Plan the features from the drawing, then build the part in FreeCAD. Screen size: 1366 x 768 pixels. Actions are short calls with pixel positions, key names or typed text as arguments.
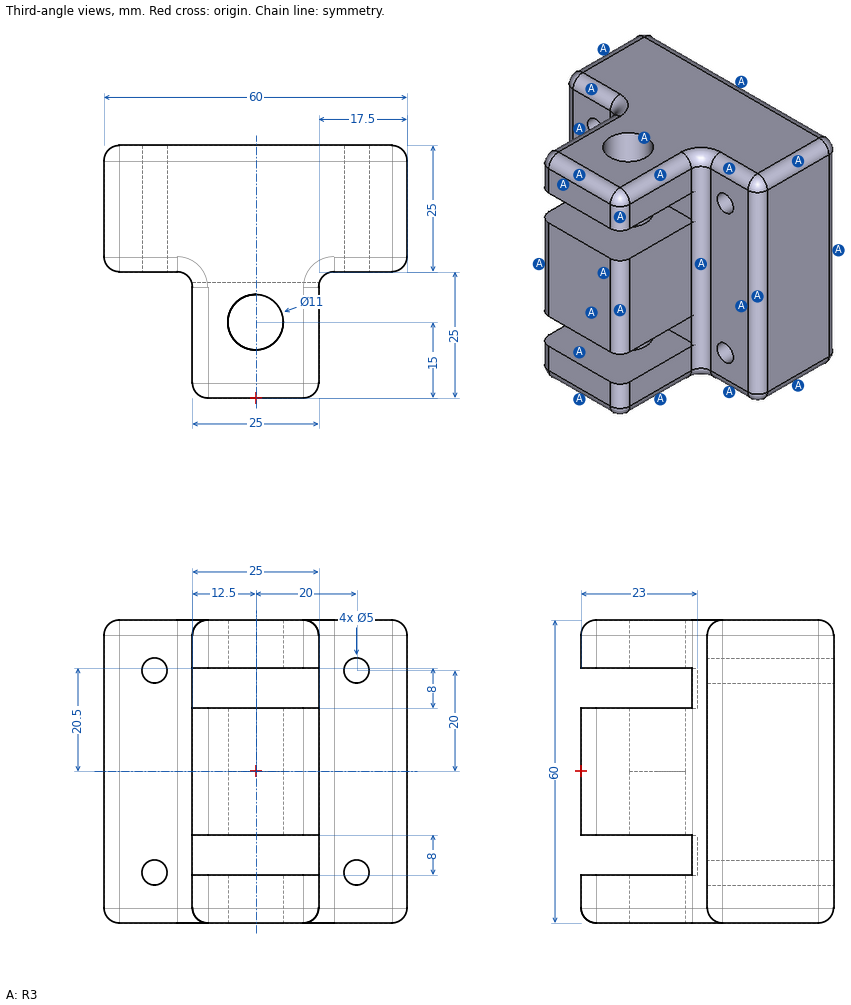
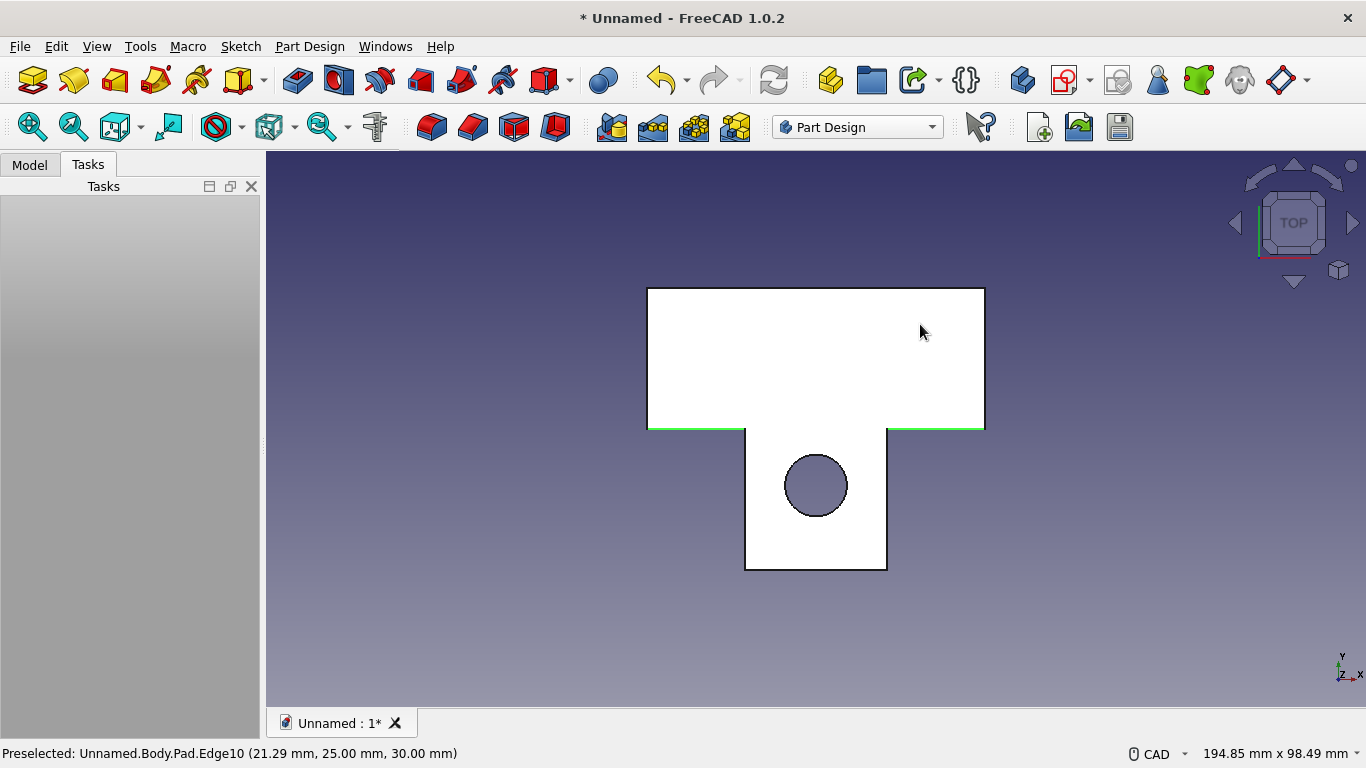
key(1)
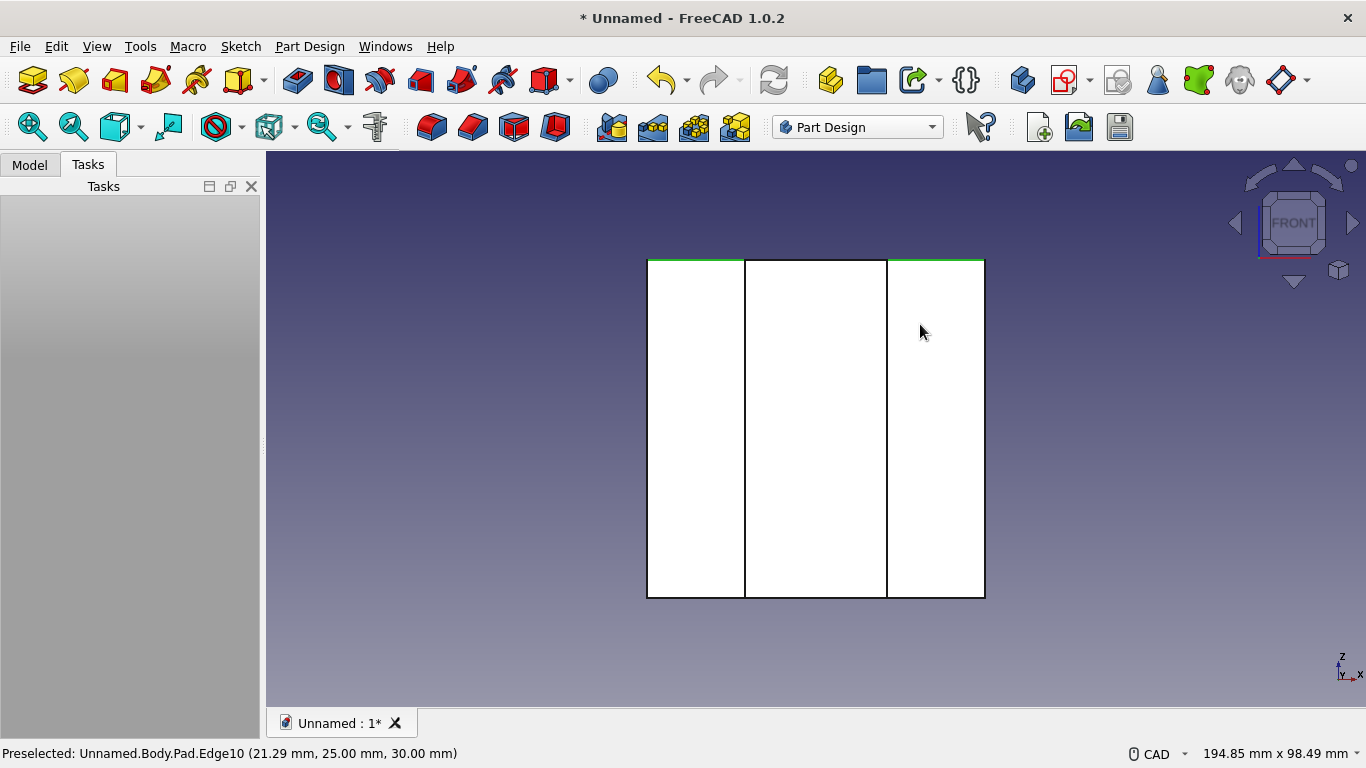
click(696, 597, ctrl)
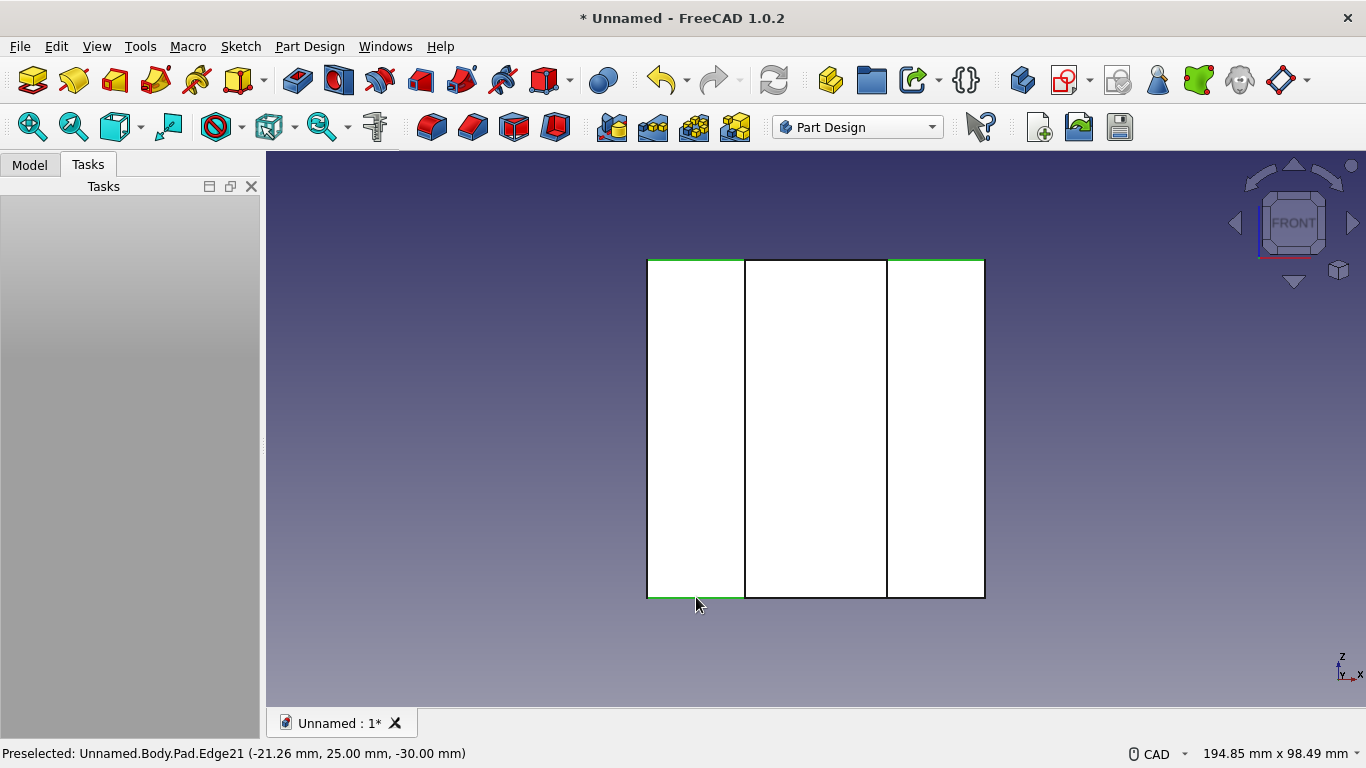
click(936, 597, ctrl)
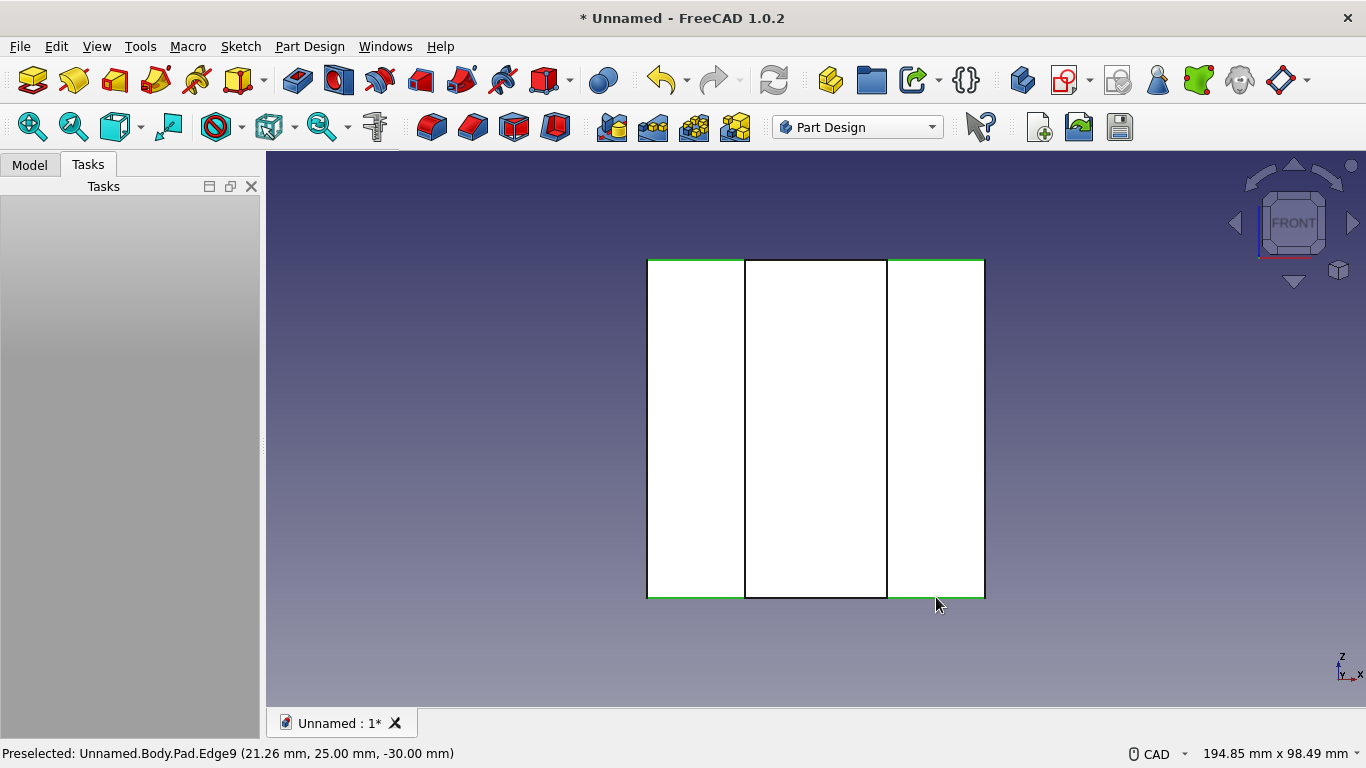
key(3)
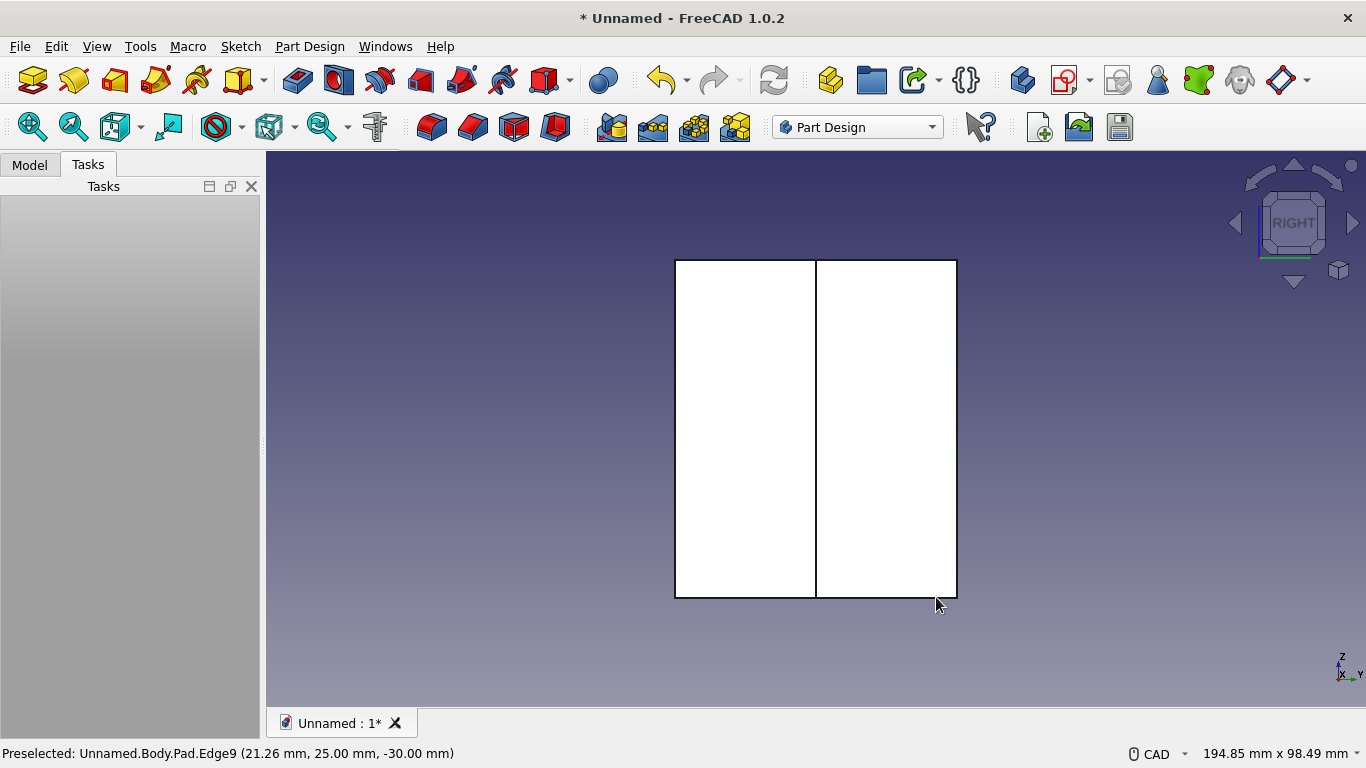
key(5)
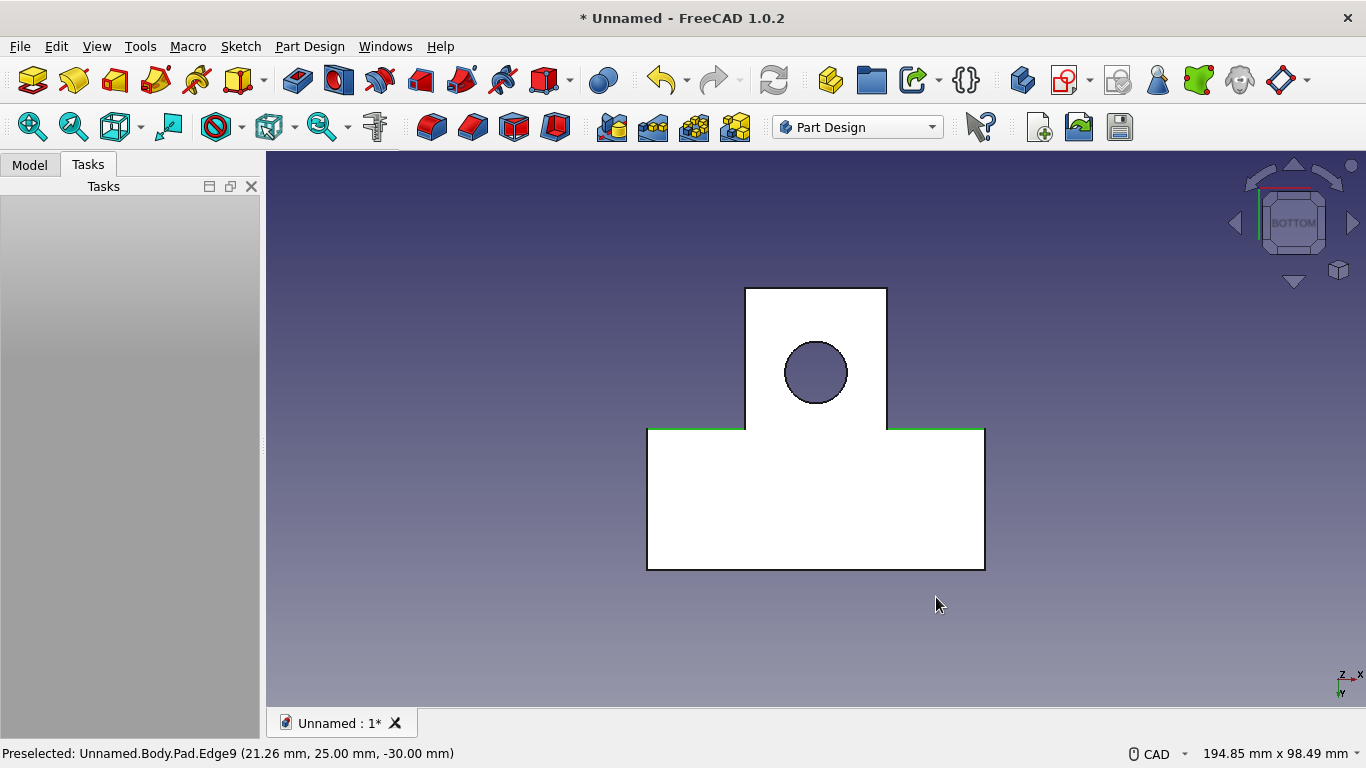
key(4)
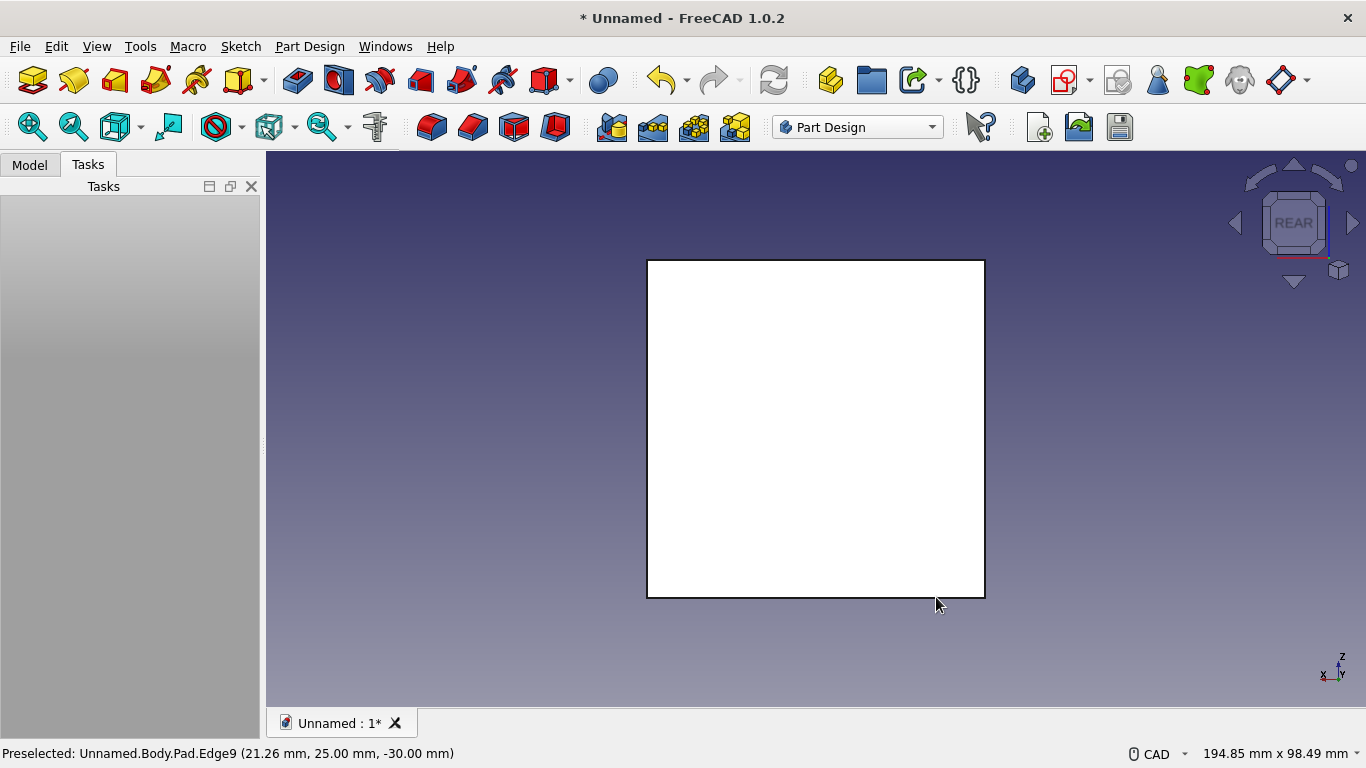
click(816, 428, ctrl)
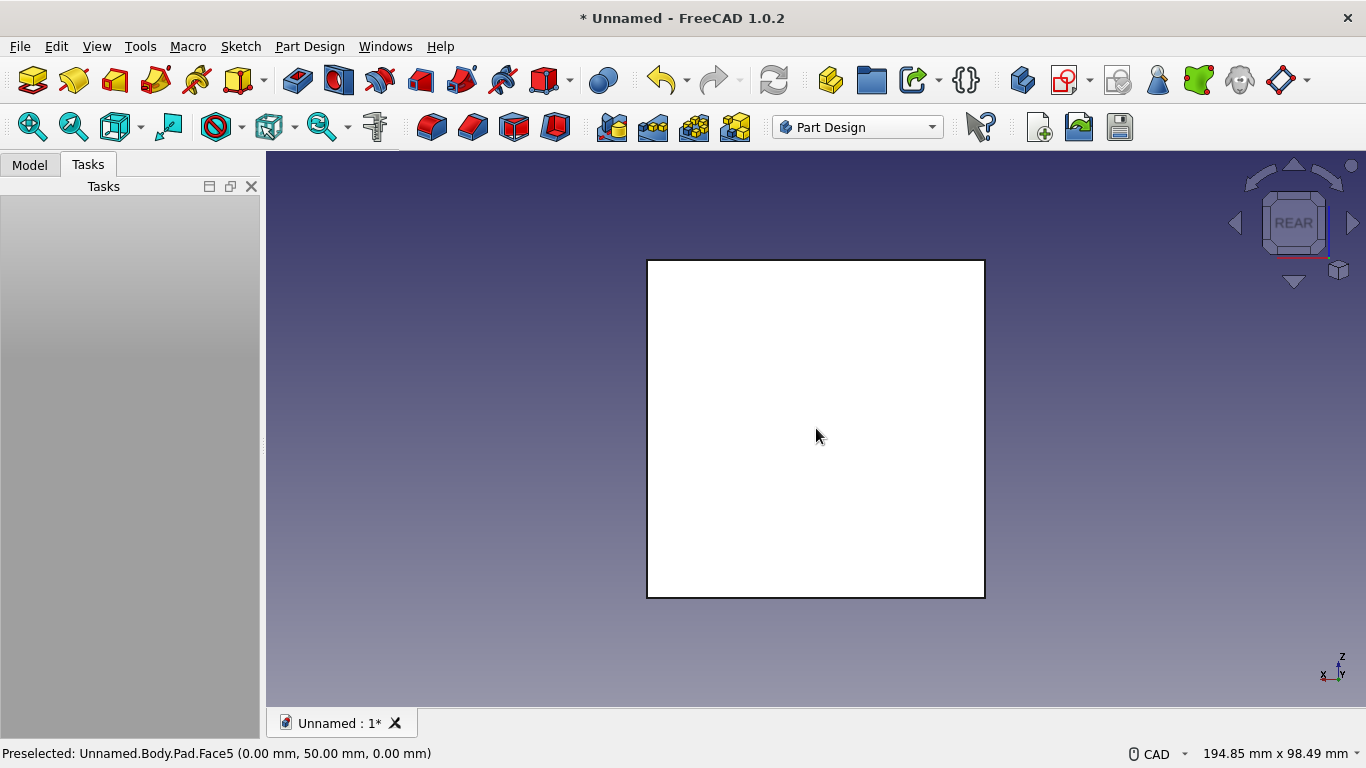
key(6)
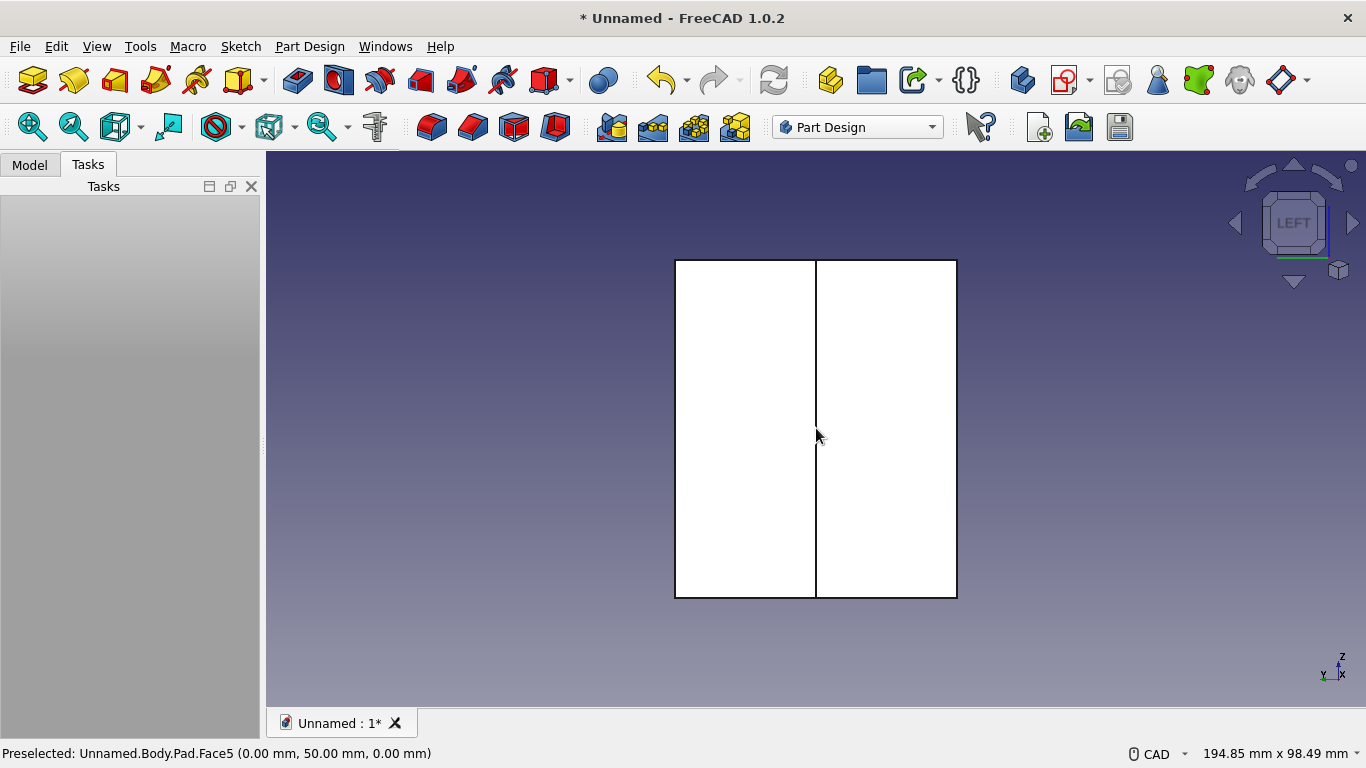
click(745, 331, ctrl)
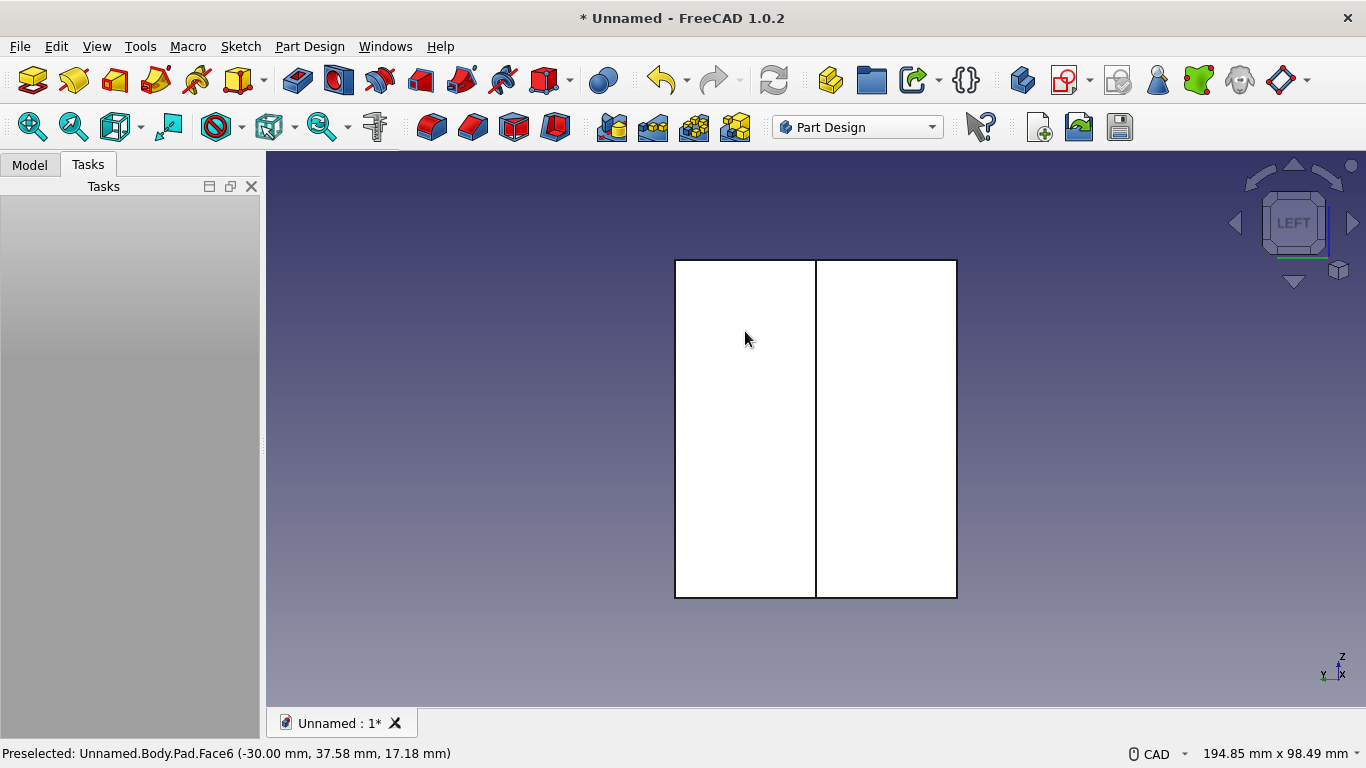
click(887, 331, ctrl)